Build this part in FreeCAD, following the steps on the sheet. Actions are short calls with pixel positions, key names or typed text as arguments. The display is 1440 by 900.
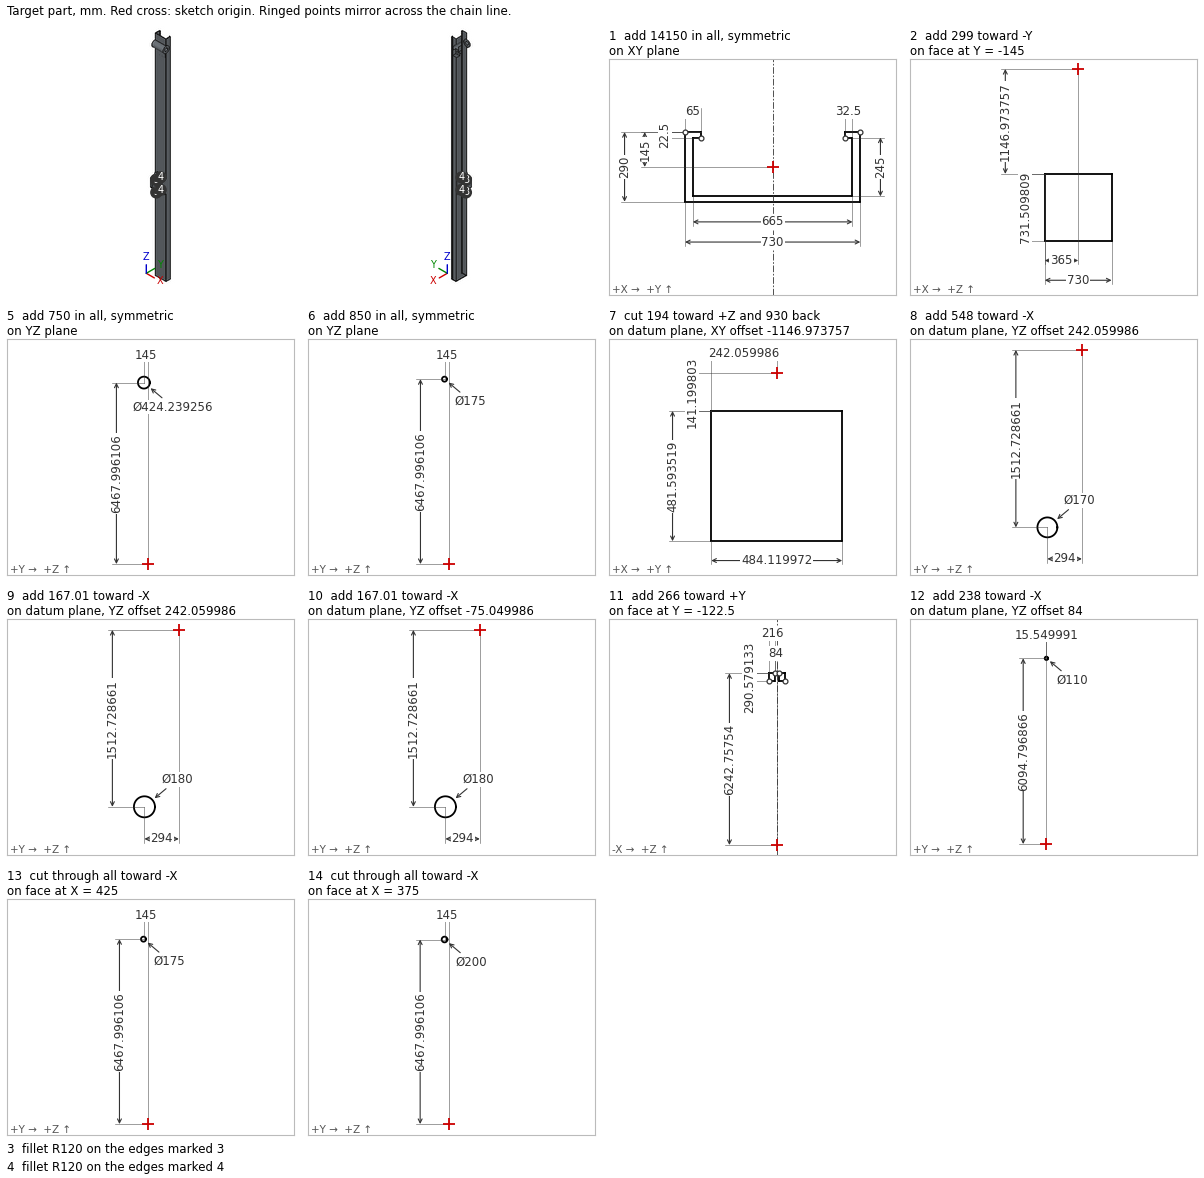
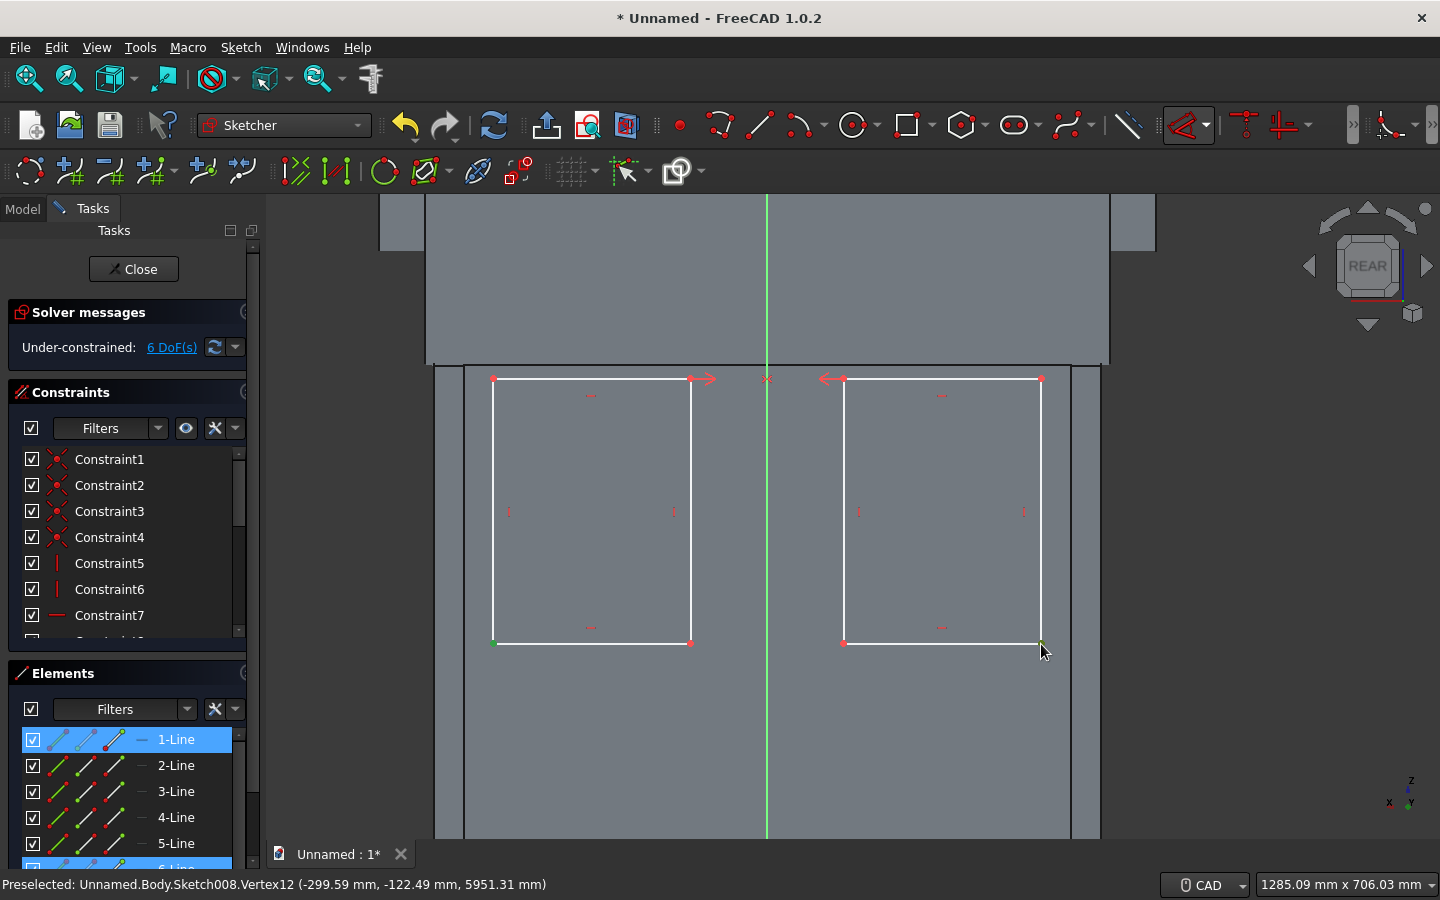
click(767, 769)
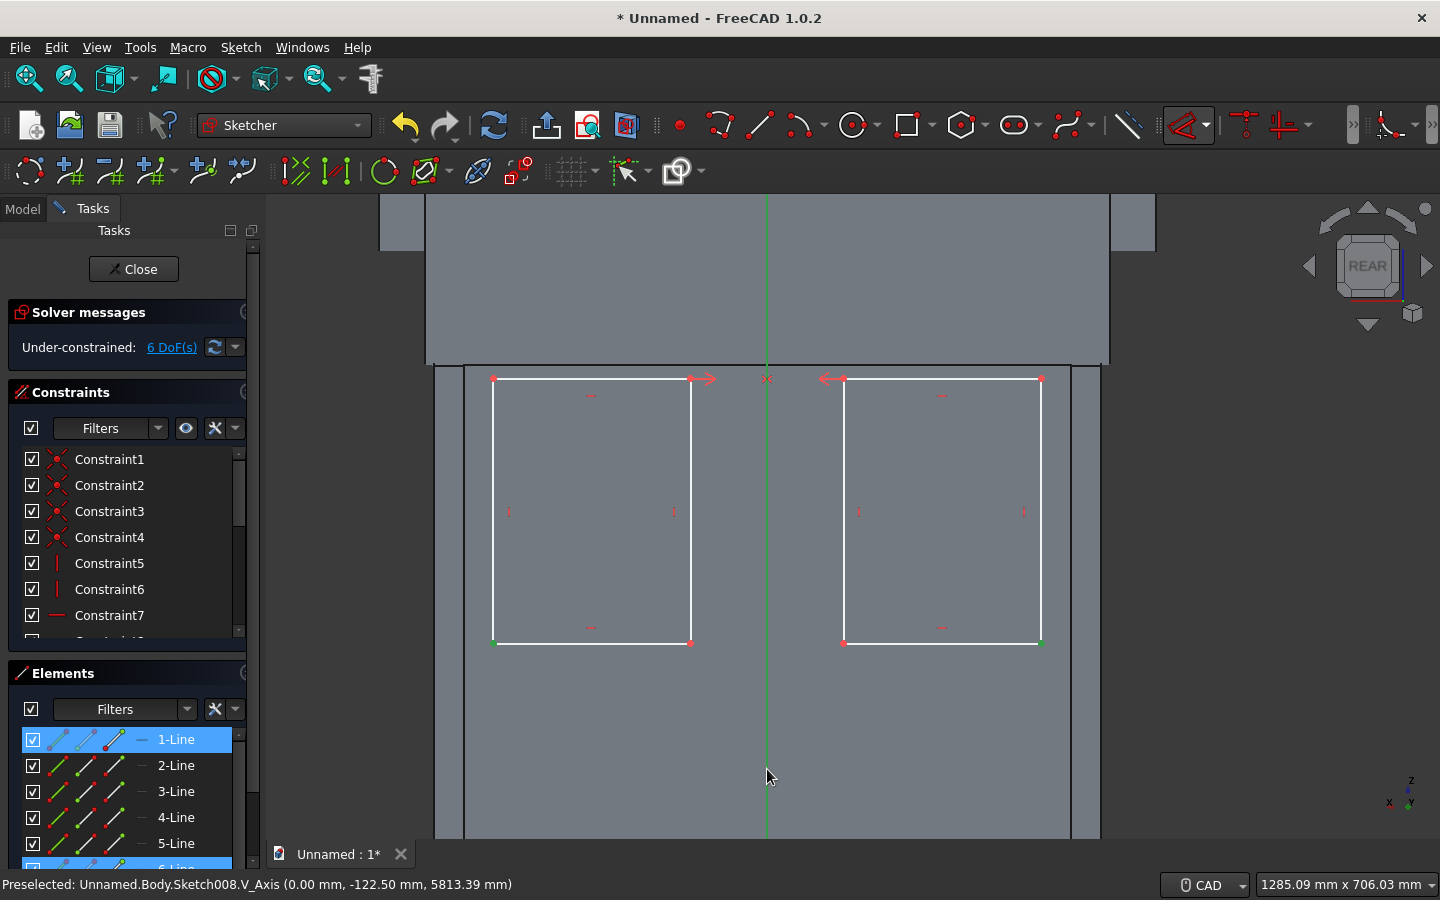
key(s)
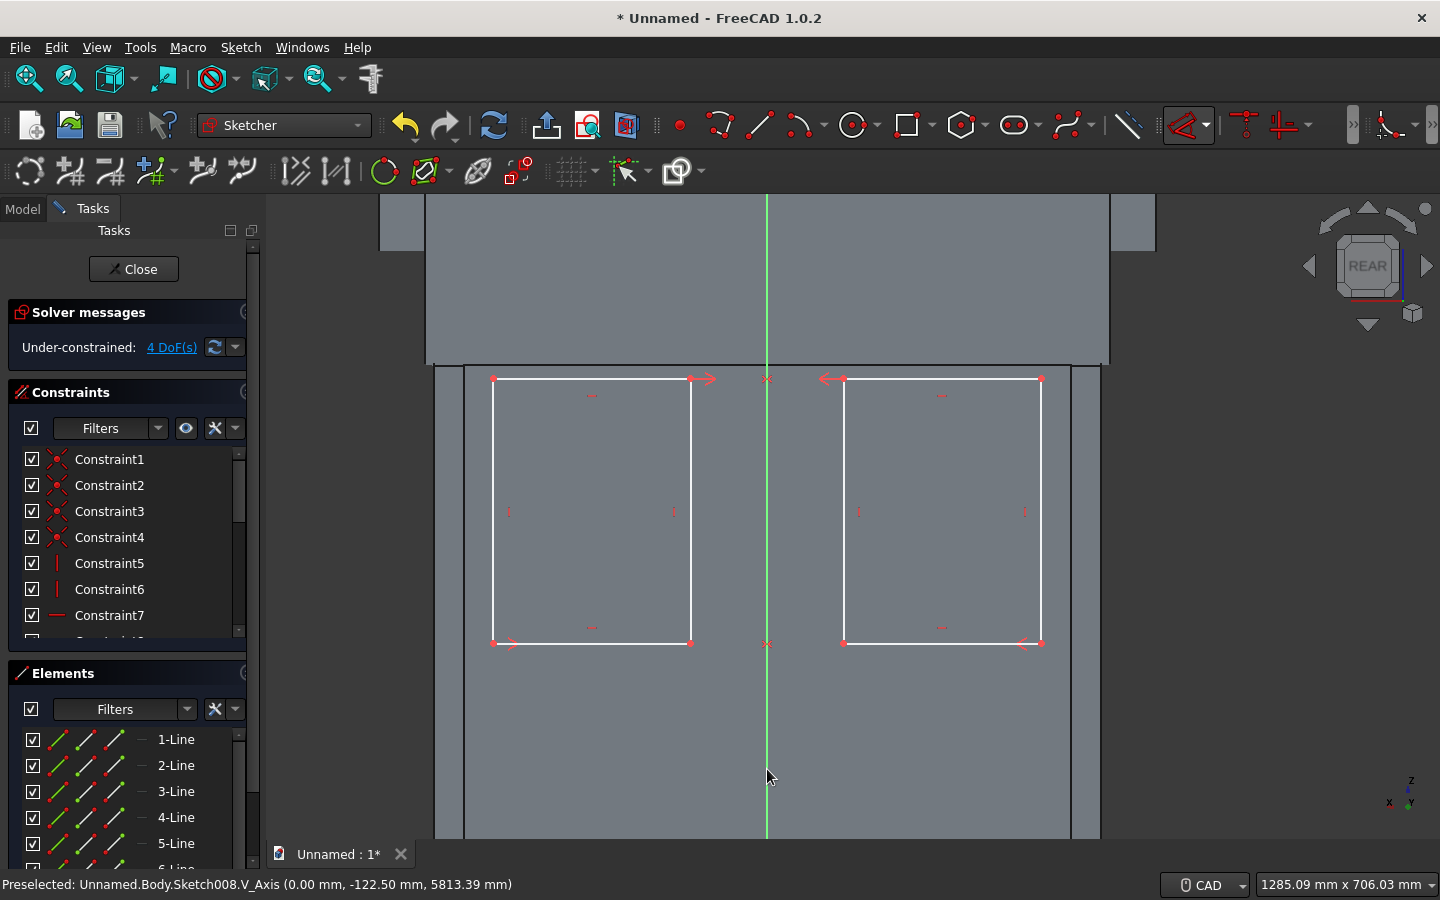
click(553, 644)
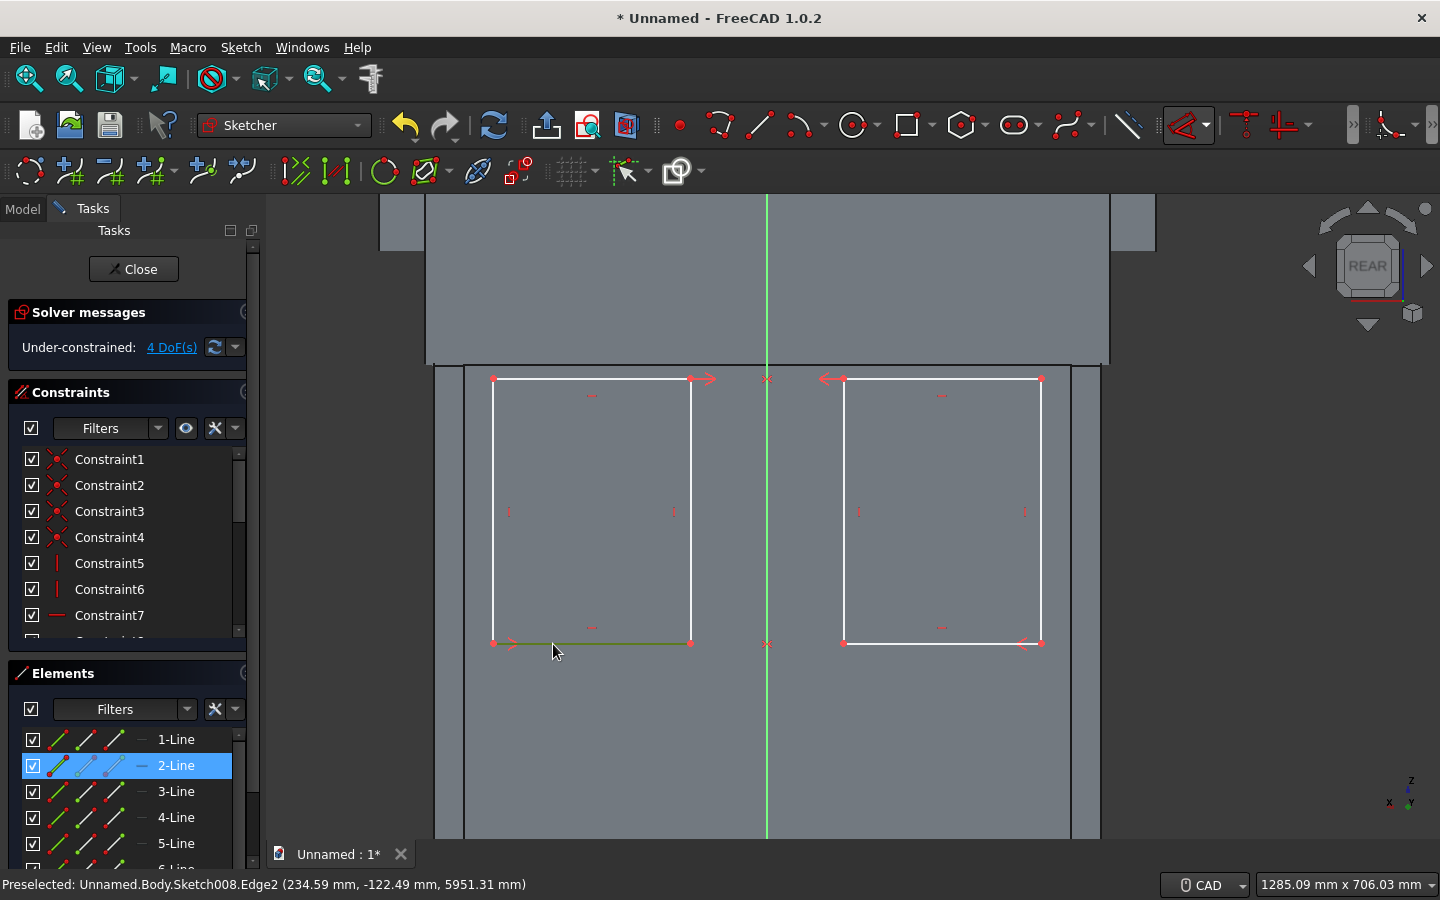
key(l)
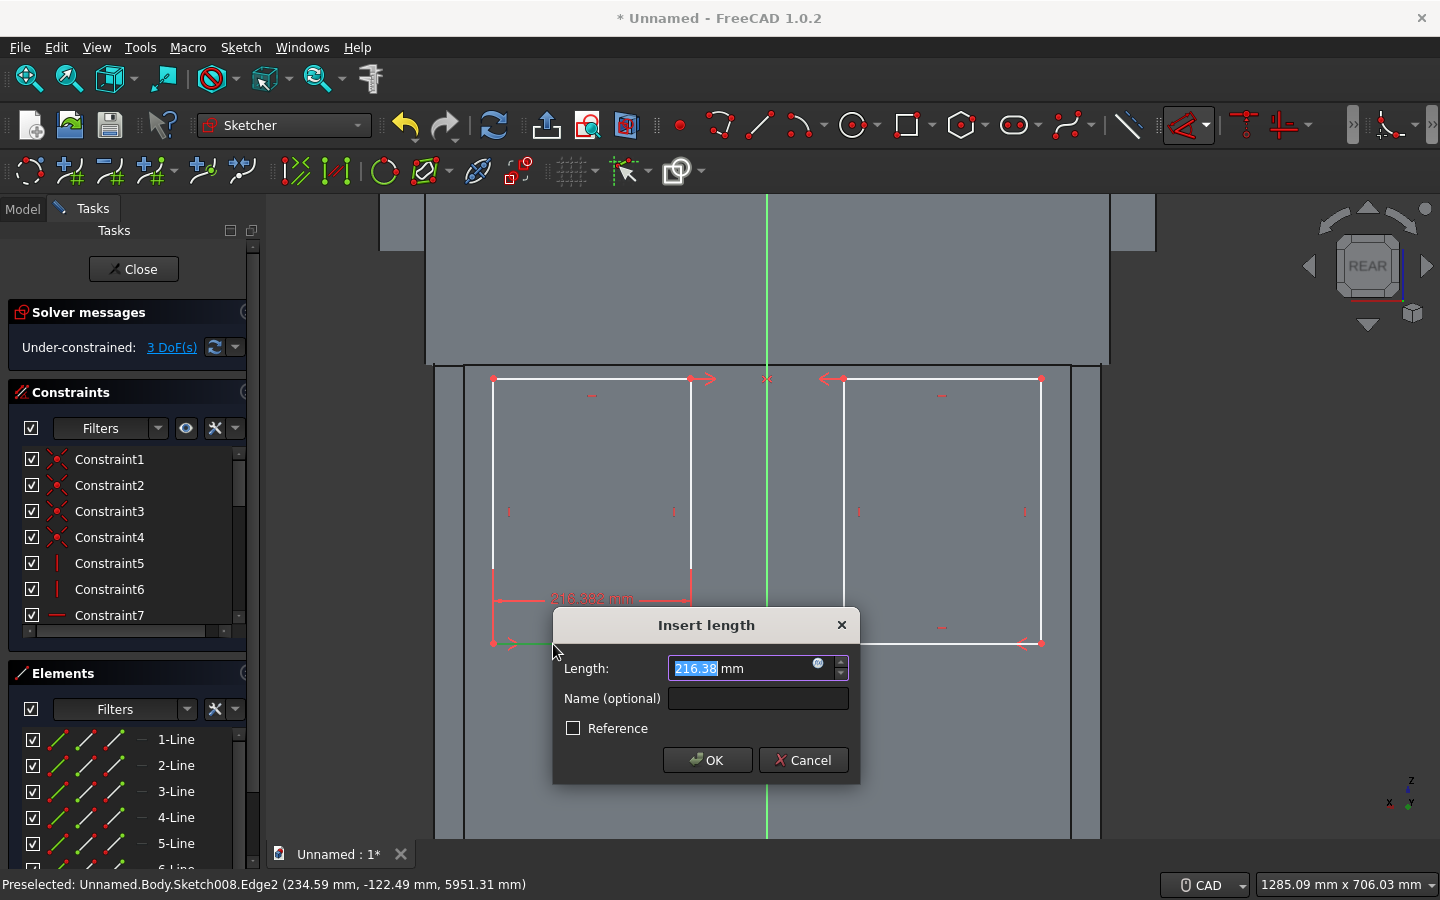
text(216)
key(Return)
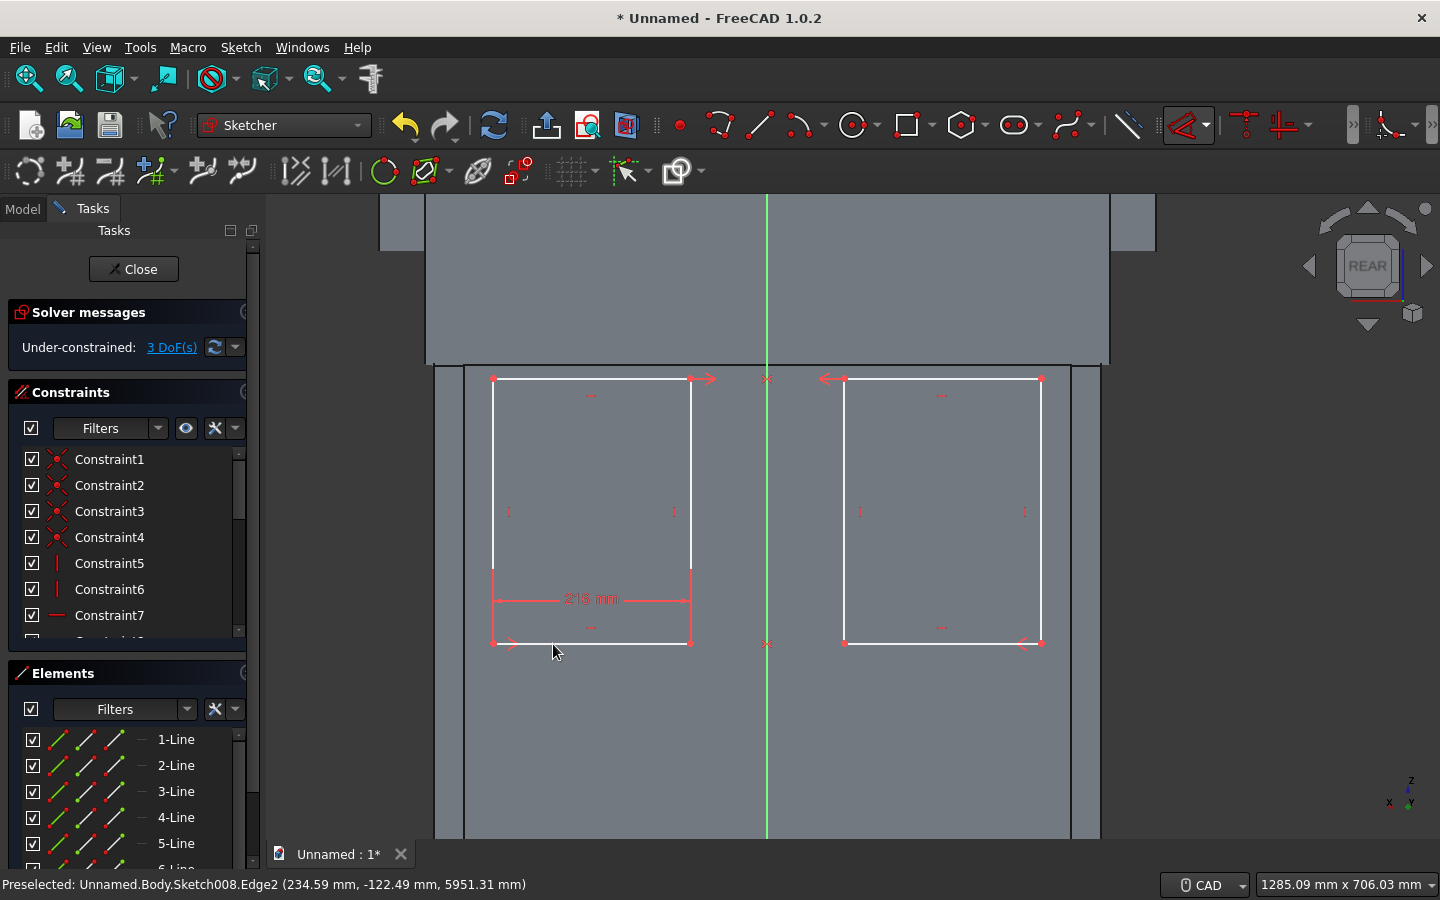
click(691, 644)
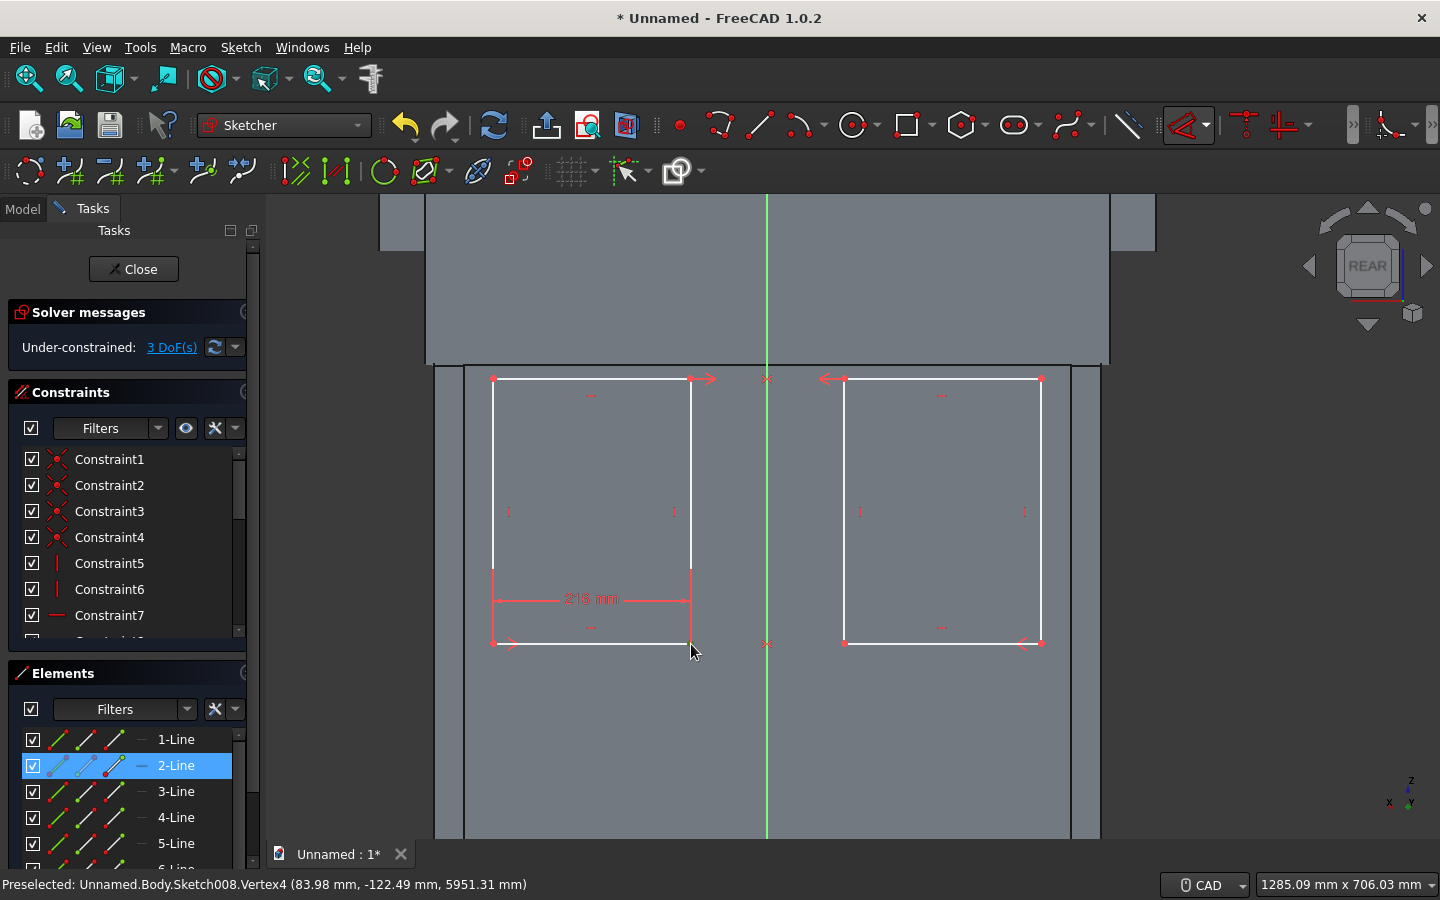
key(l)